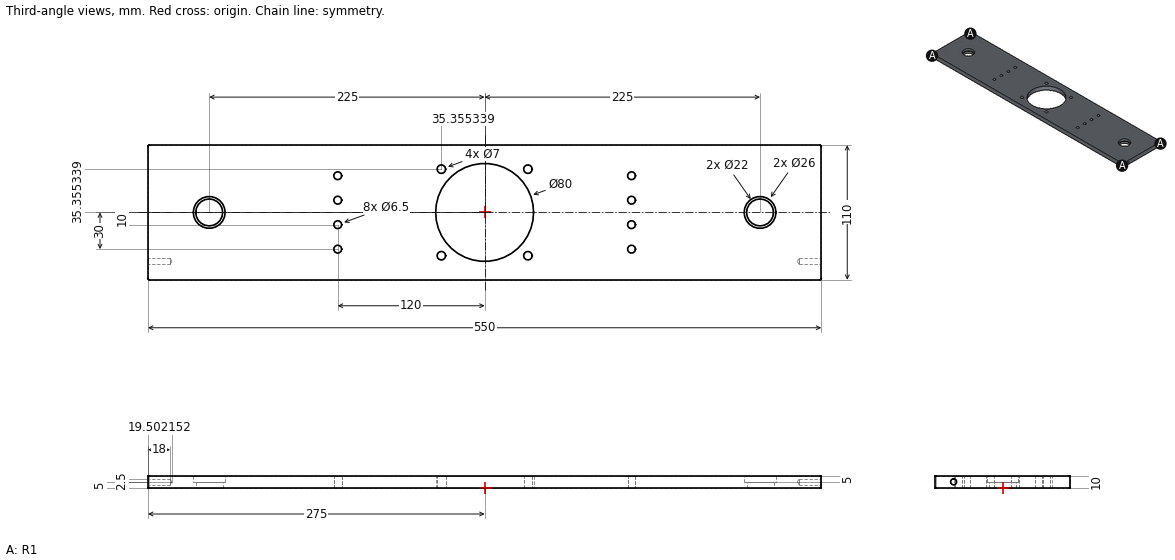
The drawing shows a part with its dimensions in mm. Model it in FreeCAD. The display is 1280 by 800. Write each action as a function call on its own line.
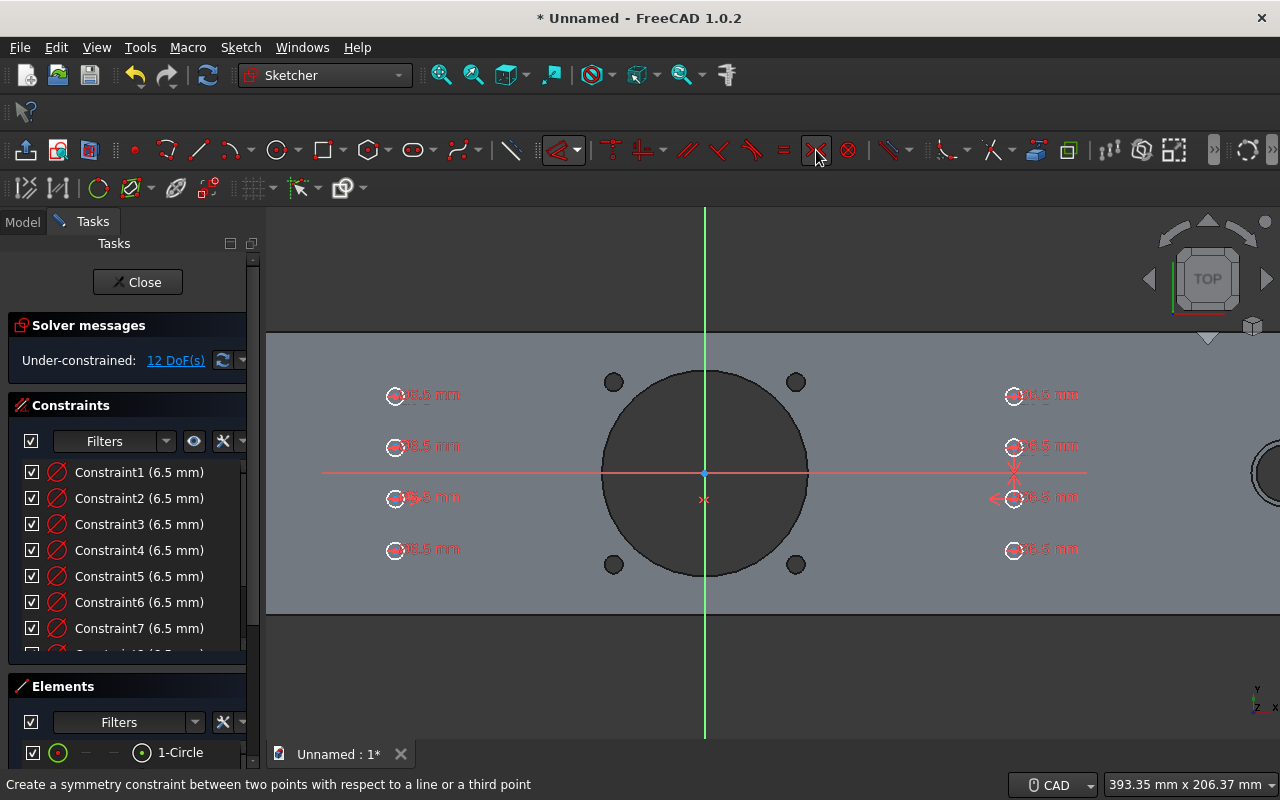
click(396, 499)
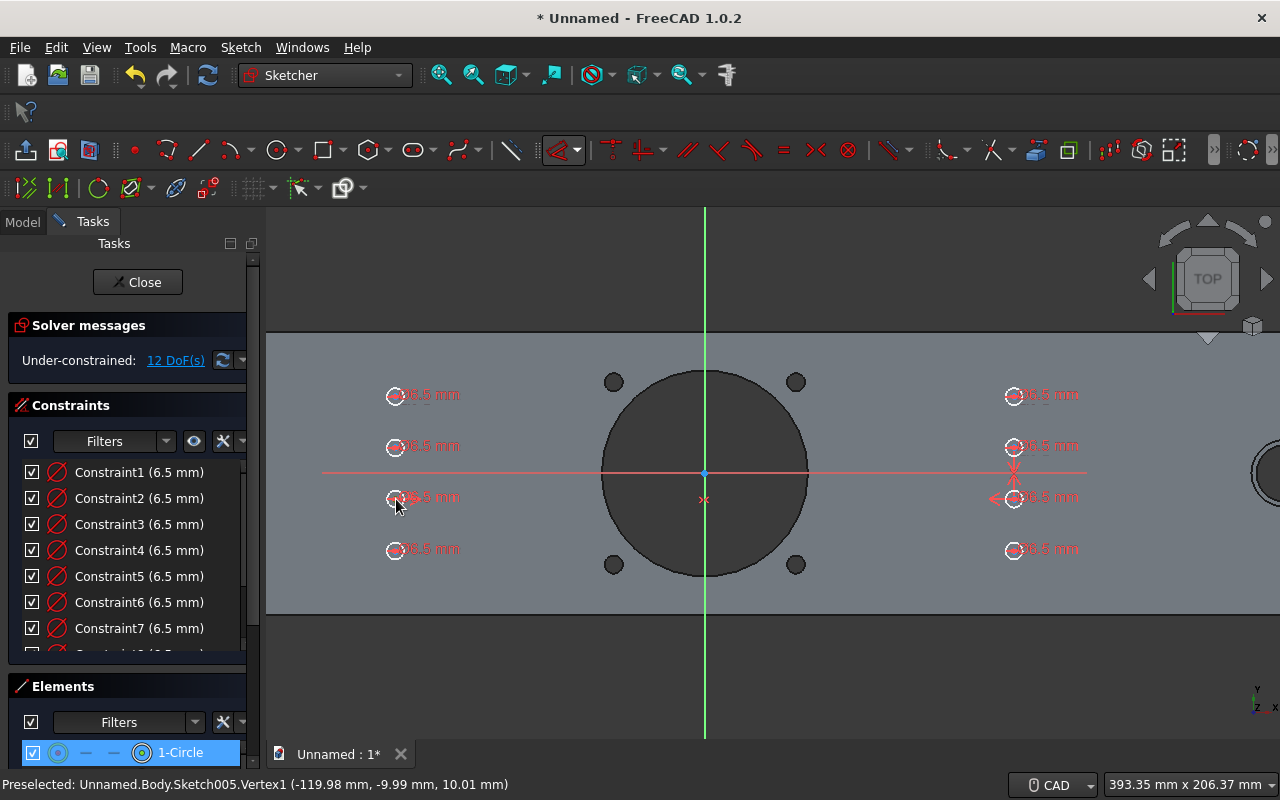
click(395, 448)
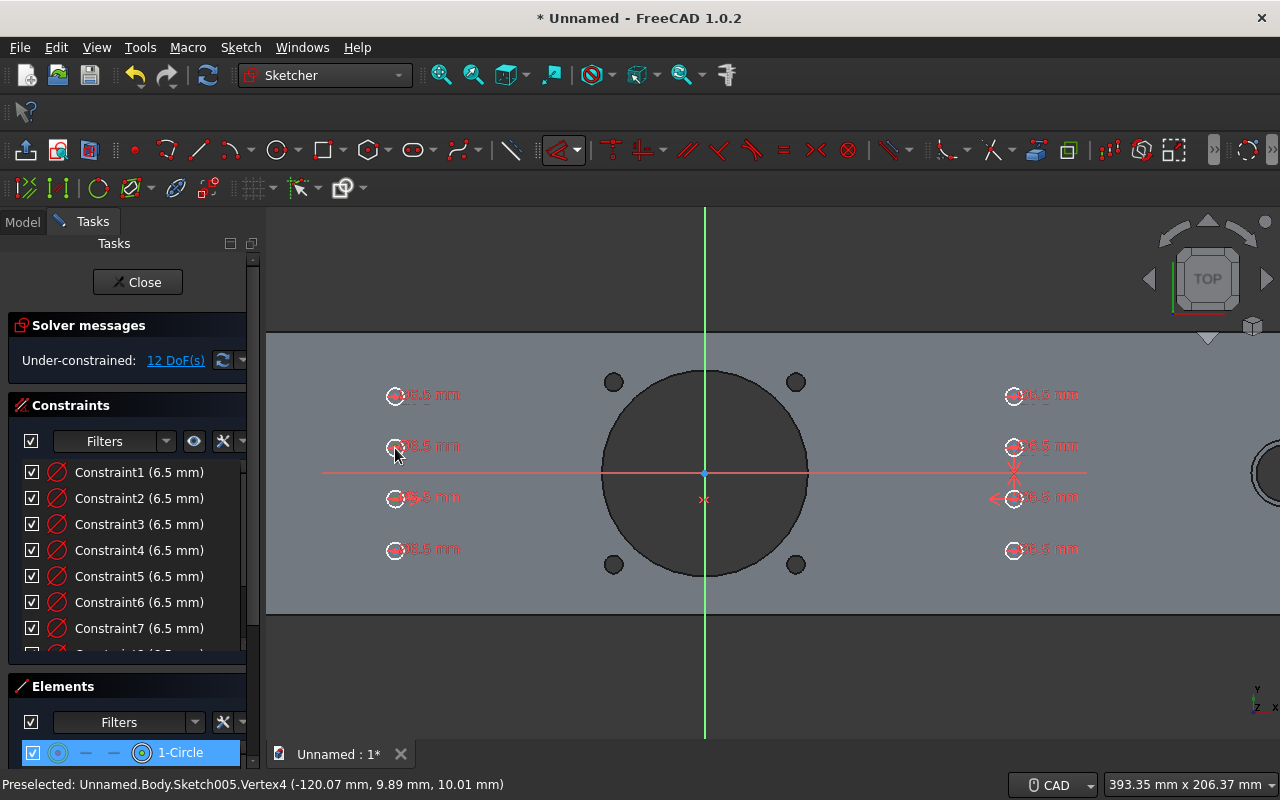
click(353, 473)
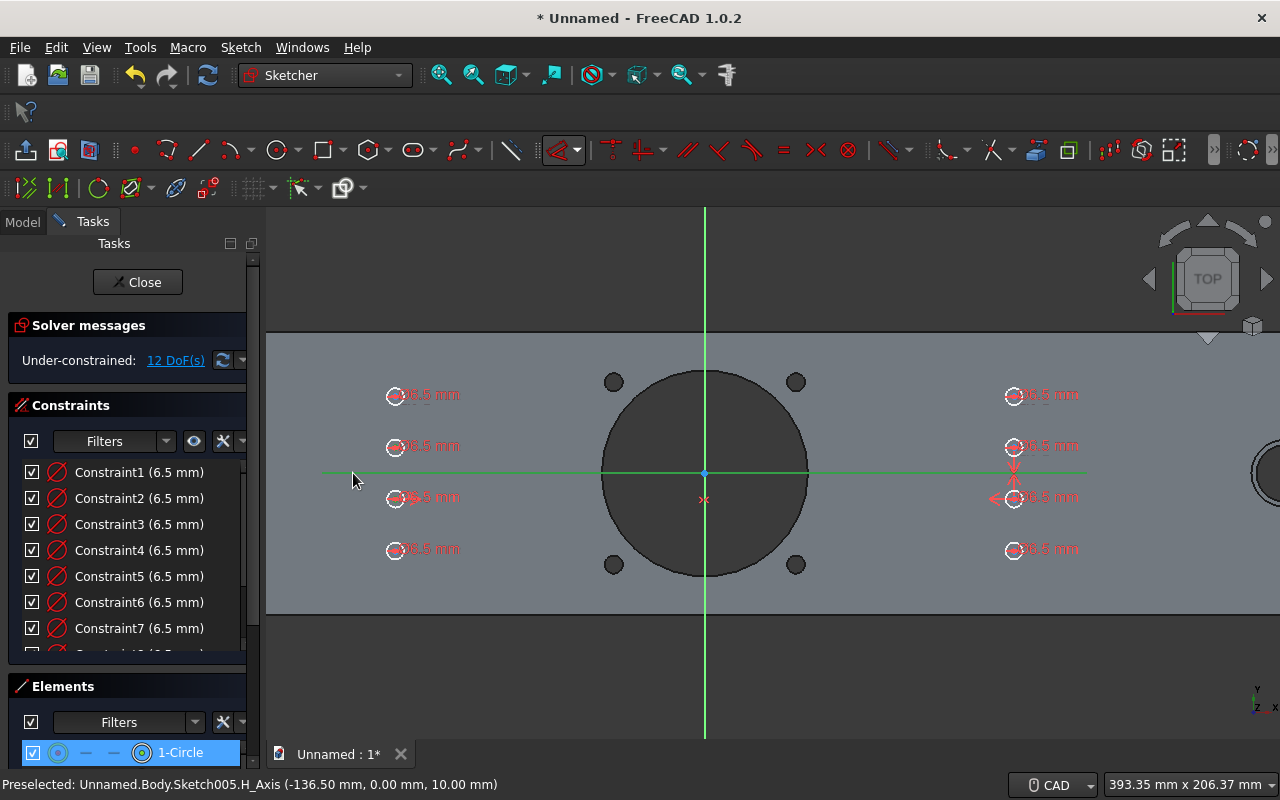
key(s)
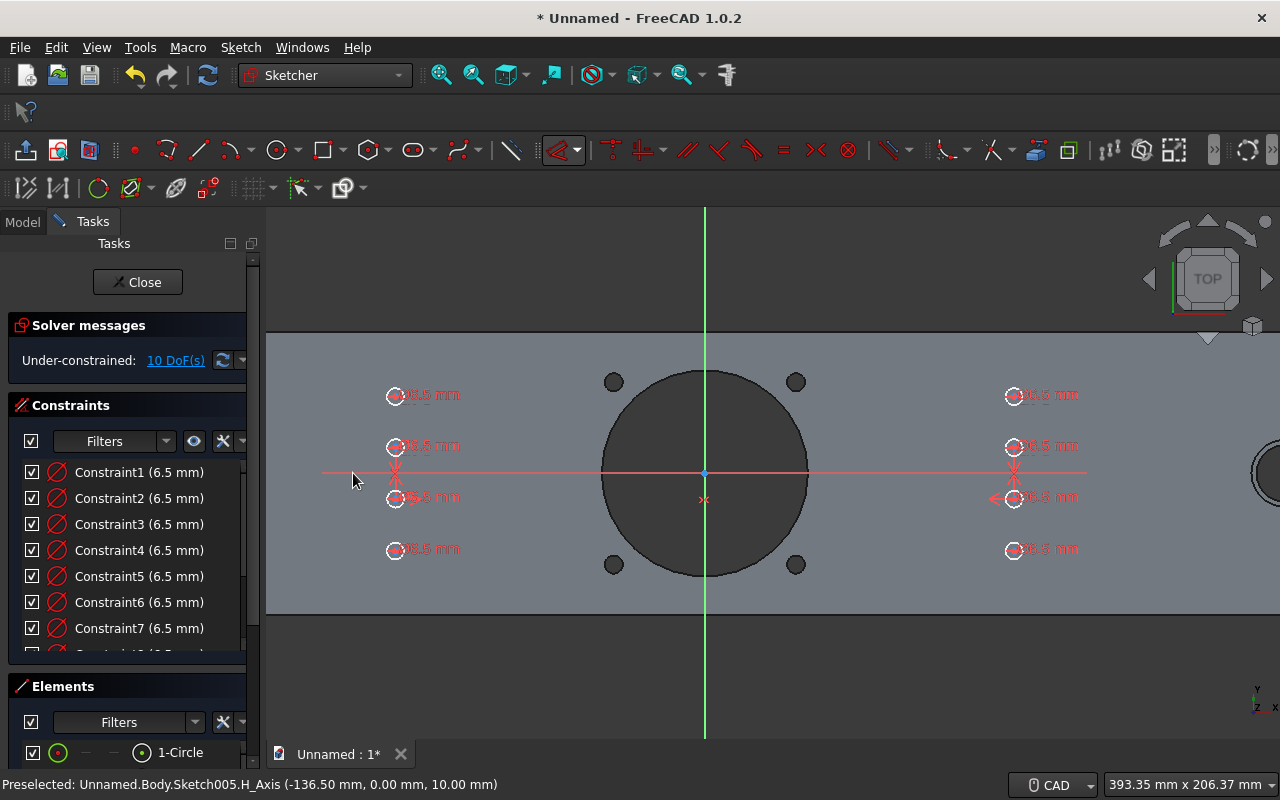
click(395, 551)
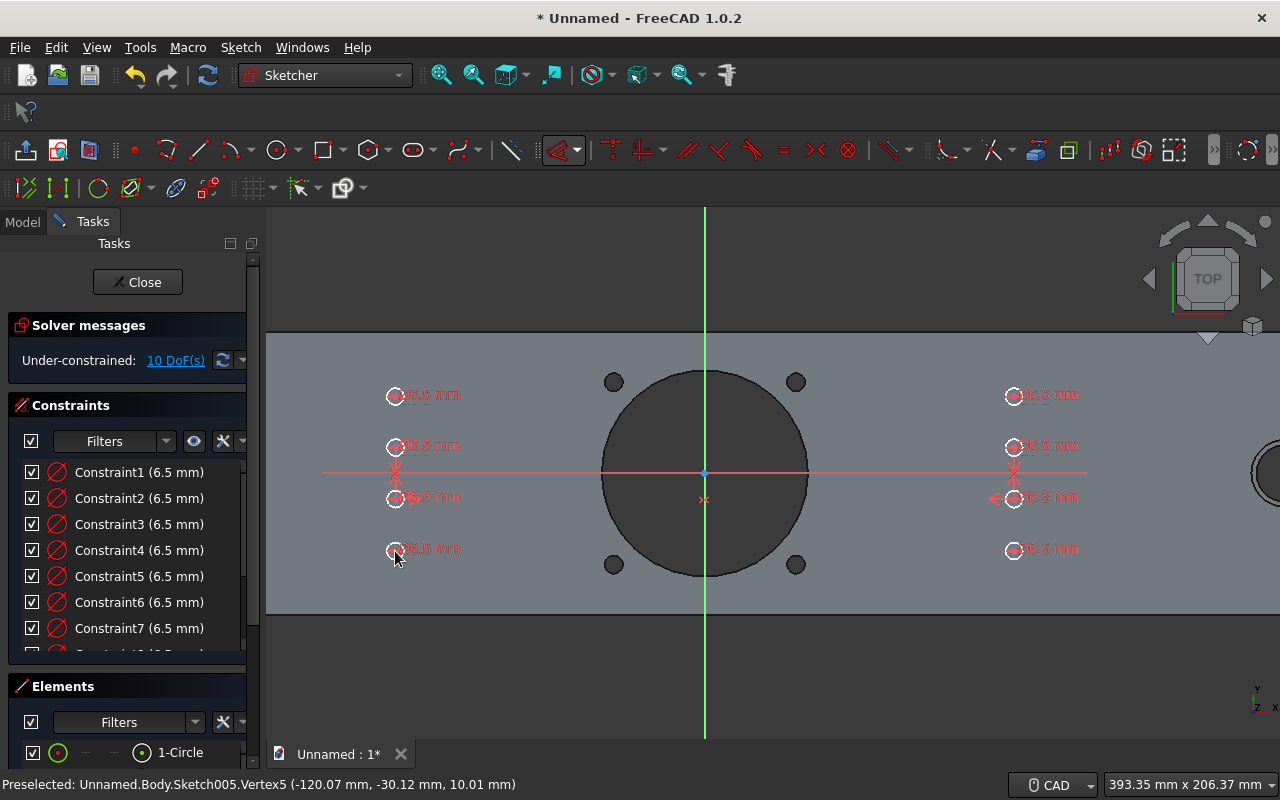
click(395, 397)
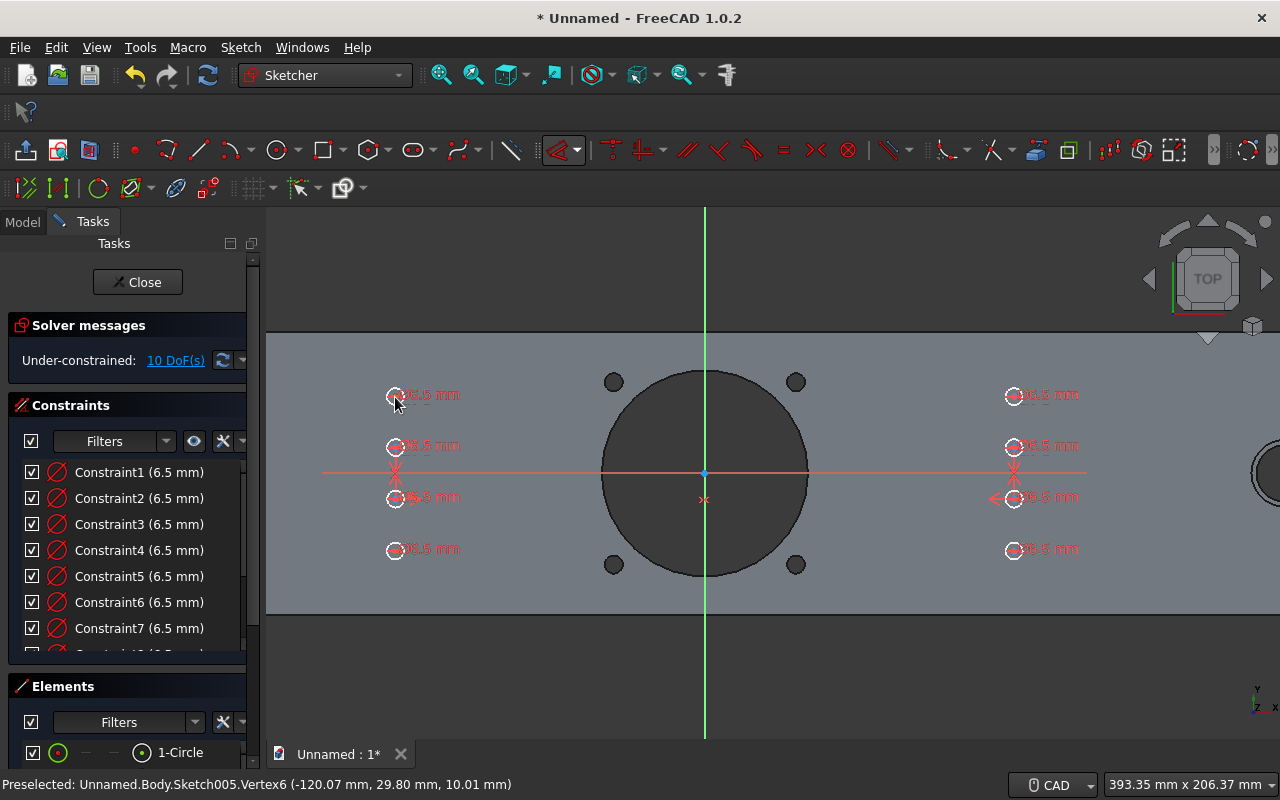
click(353, 473)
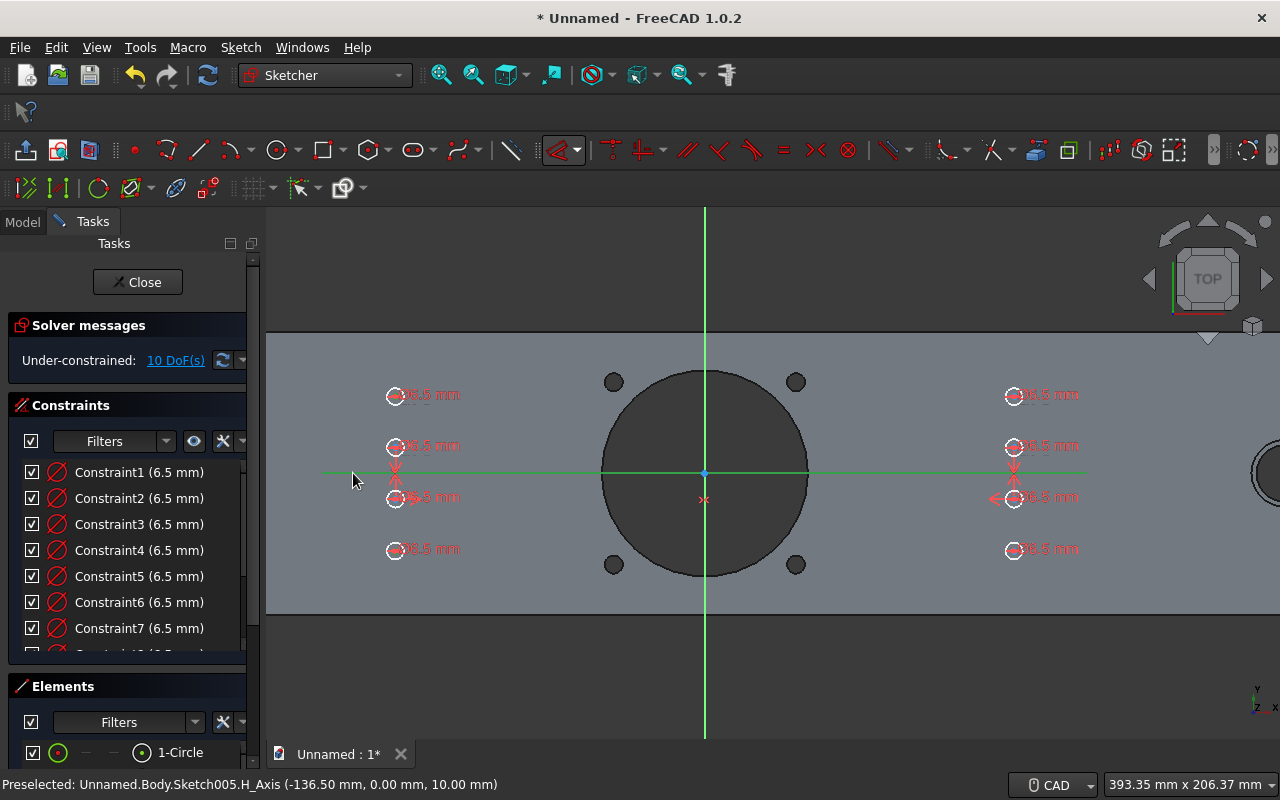
key(s)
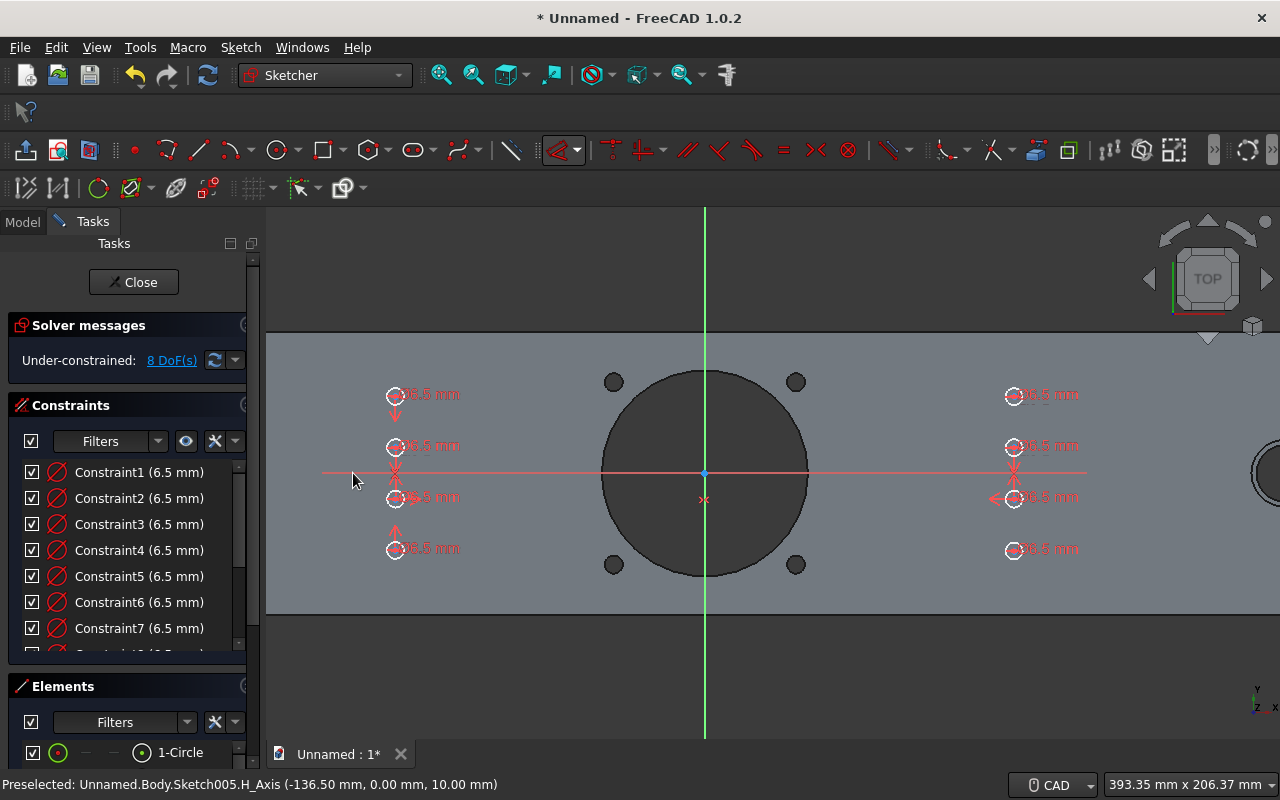
click(395, 396)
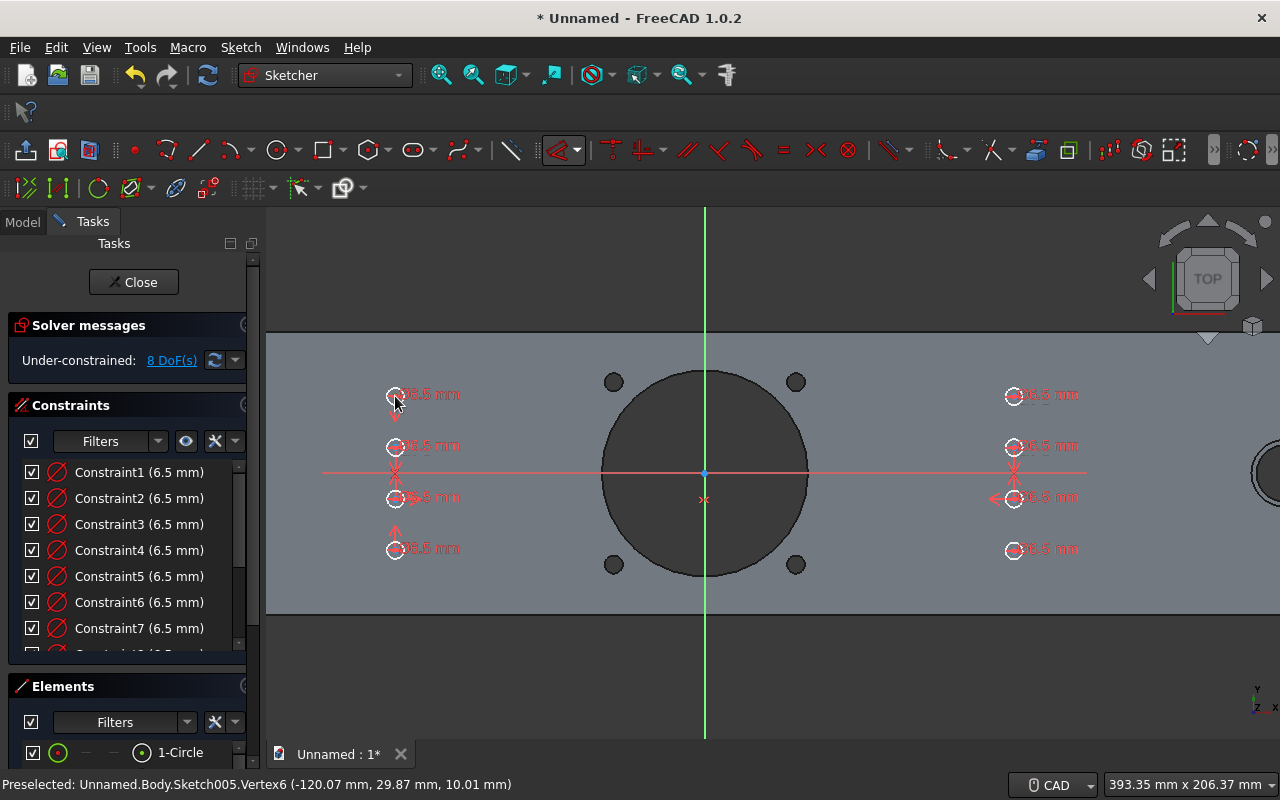
click(1014, 397)